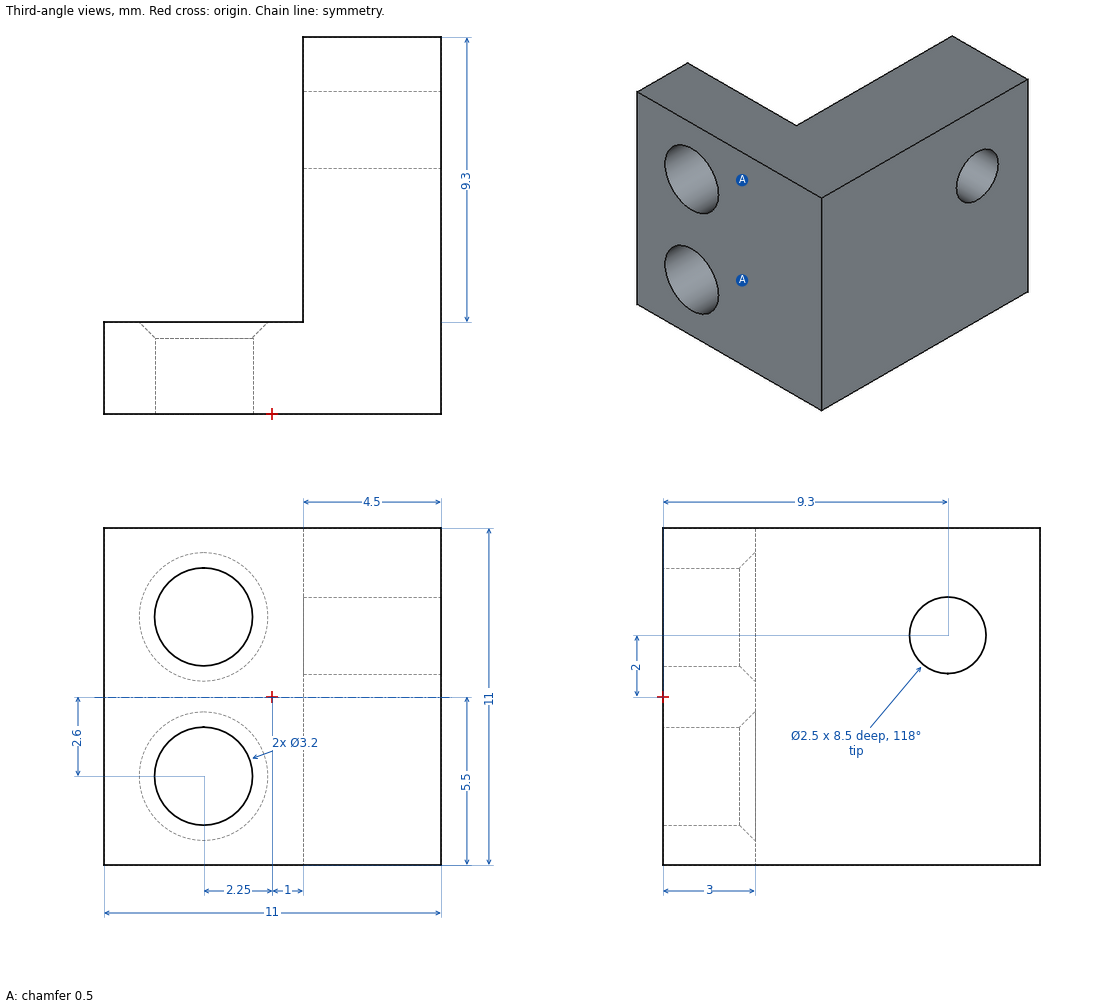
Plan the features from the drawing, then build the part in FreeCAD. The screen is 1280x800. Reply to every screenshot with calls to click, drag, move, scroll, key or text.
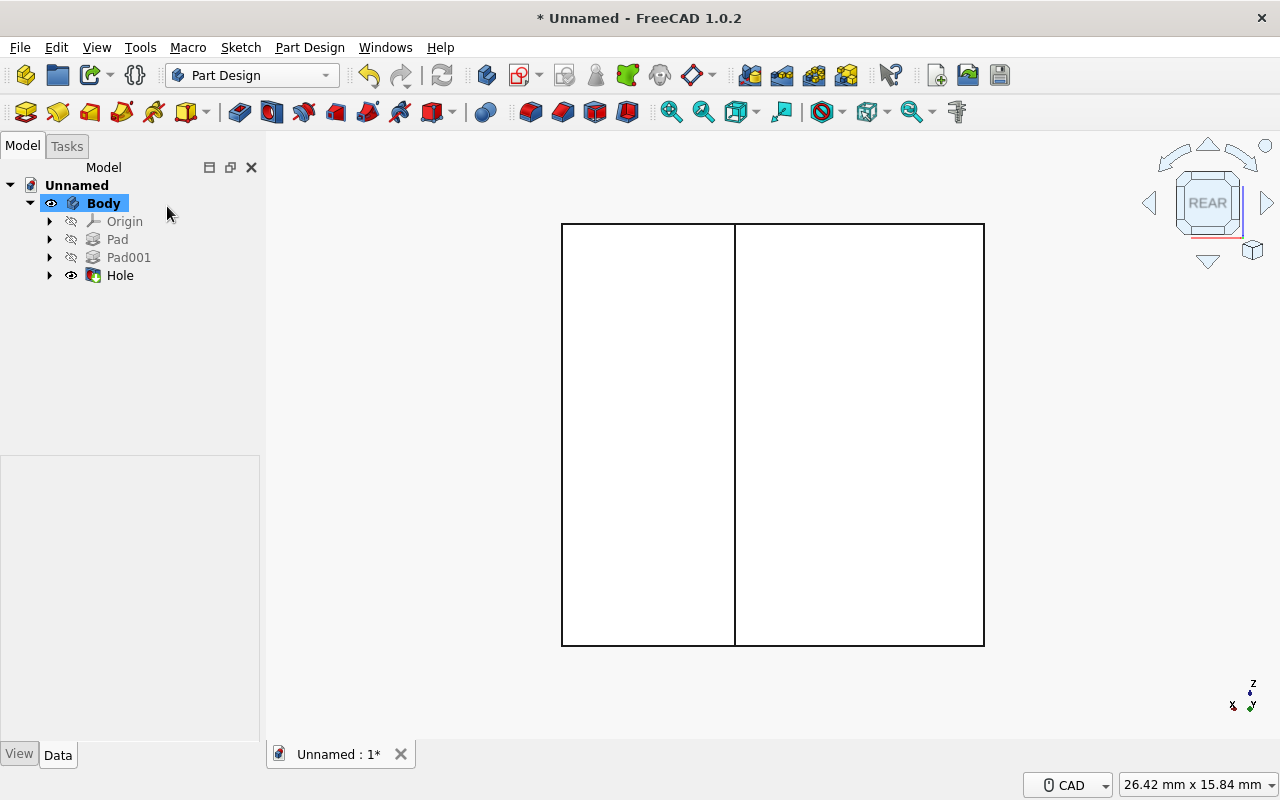
click(859, 374)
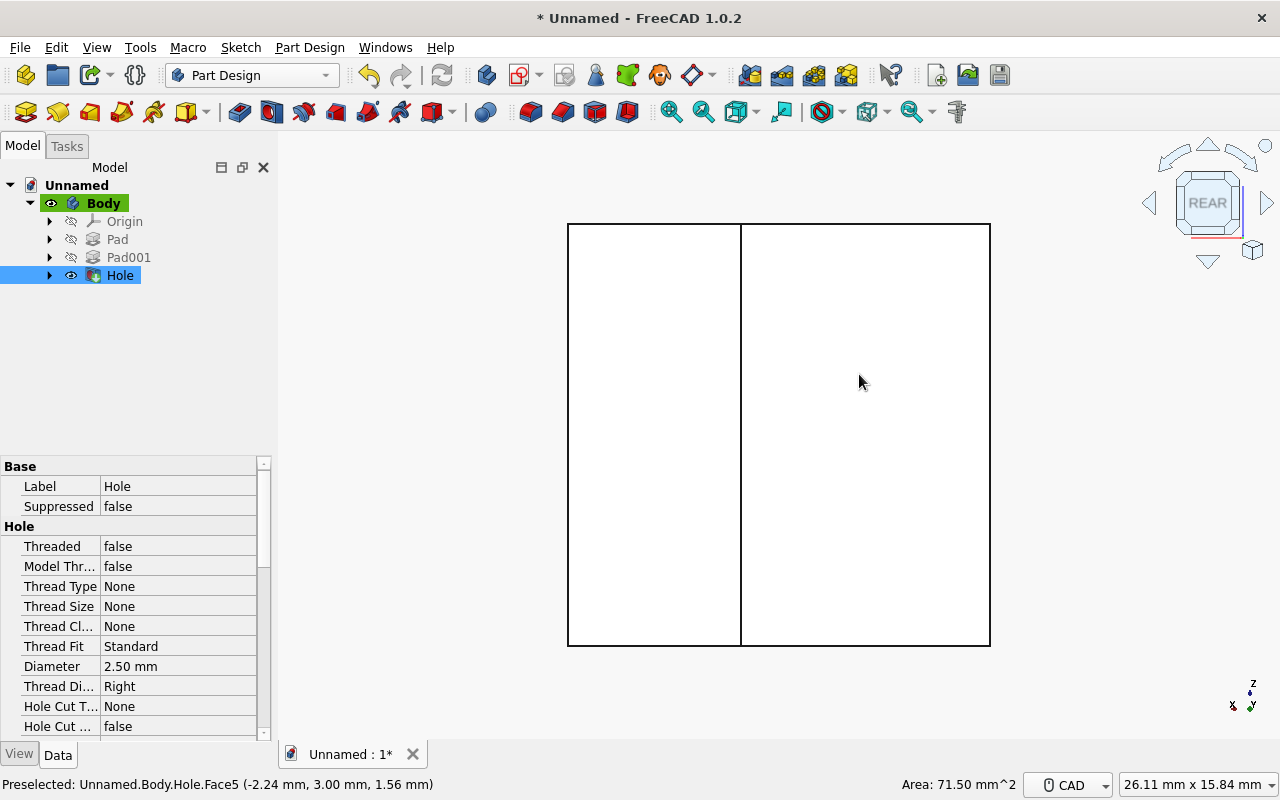
click(520, 76)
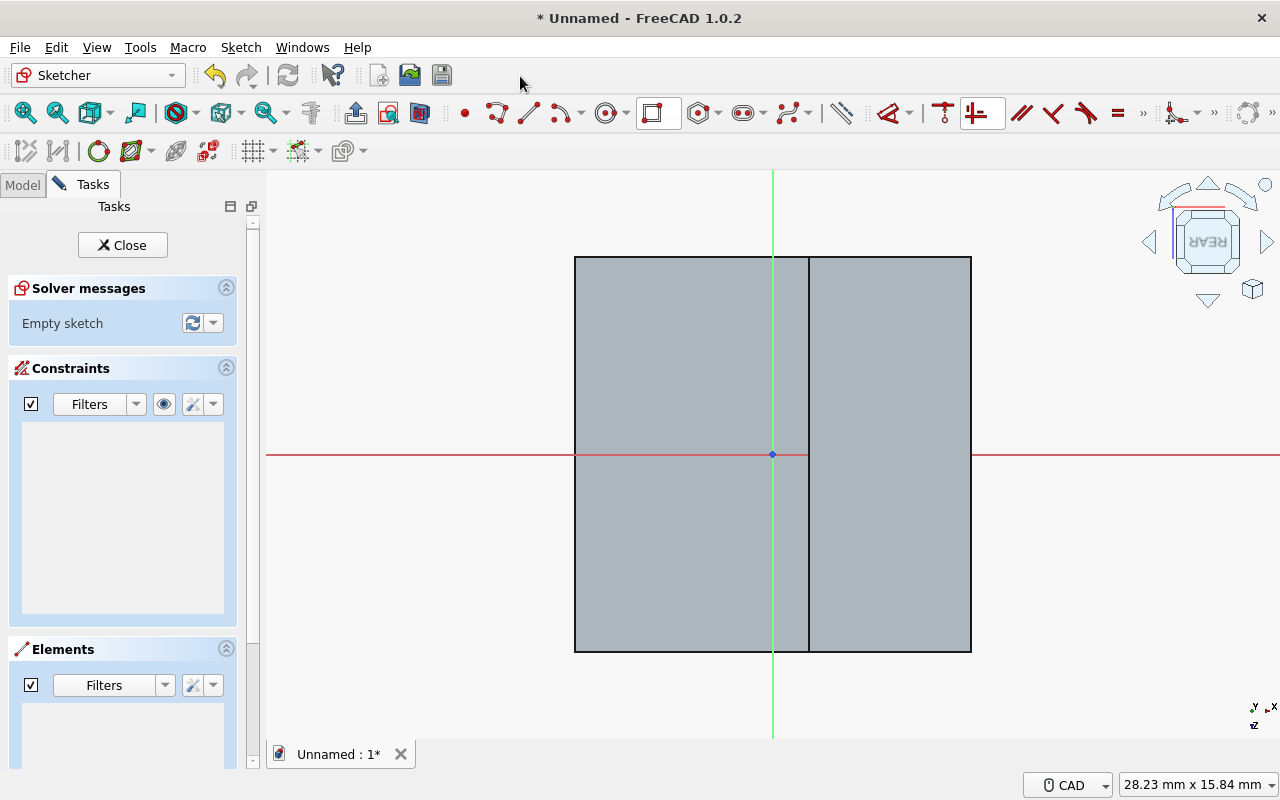
click(606, 114)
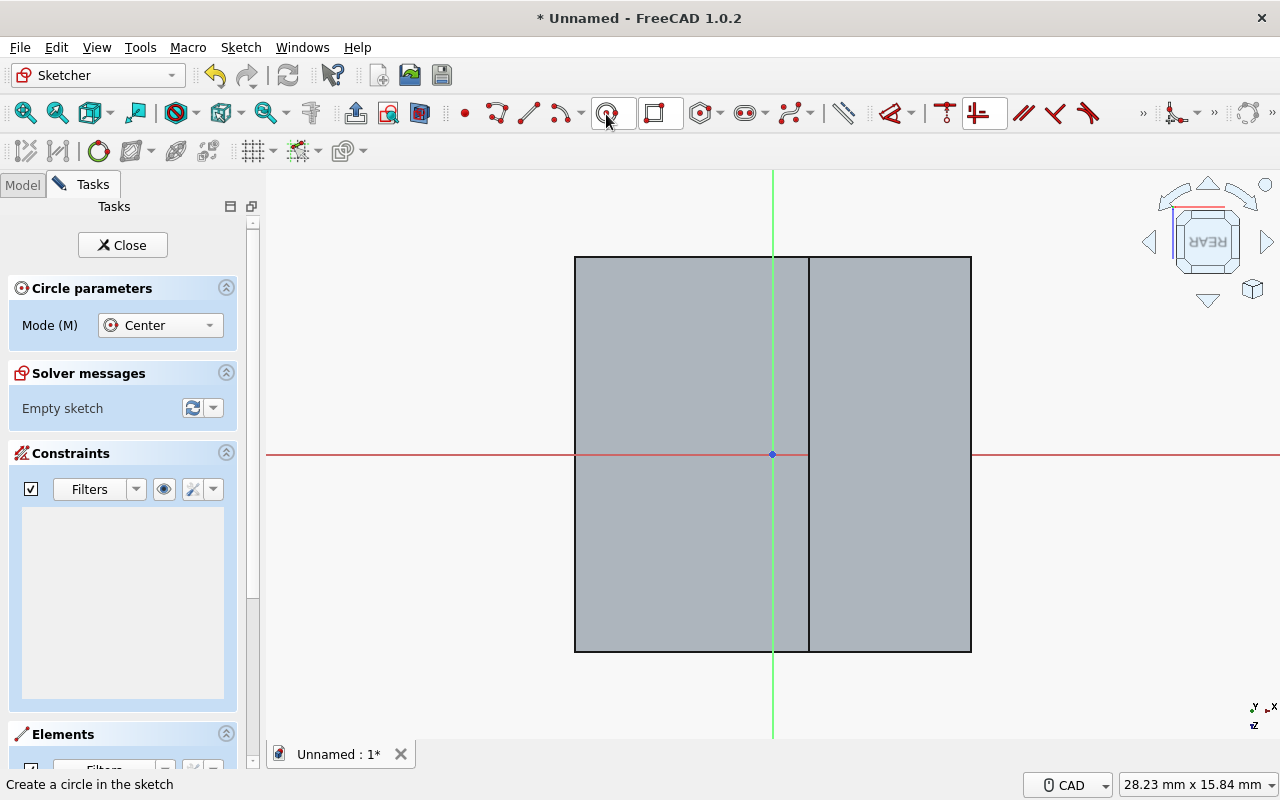
click(692, 361)
click(733, 320)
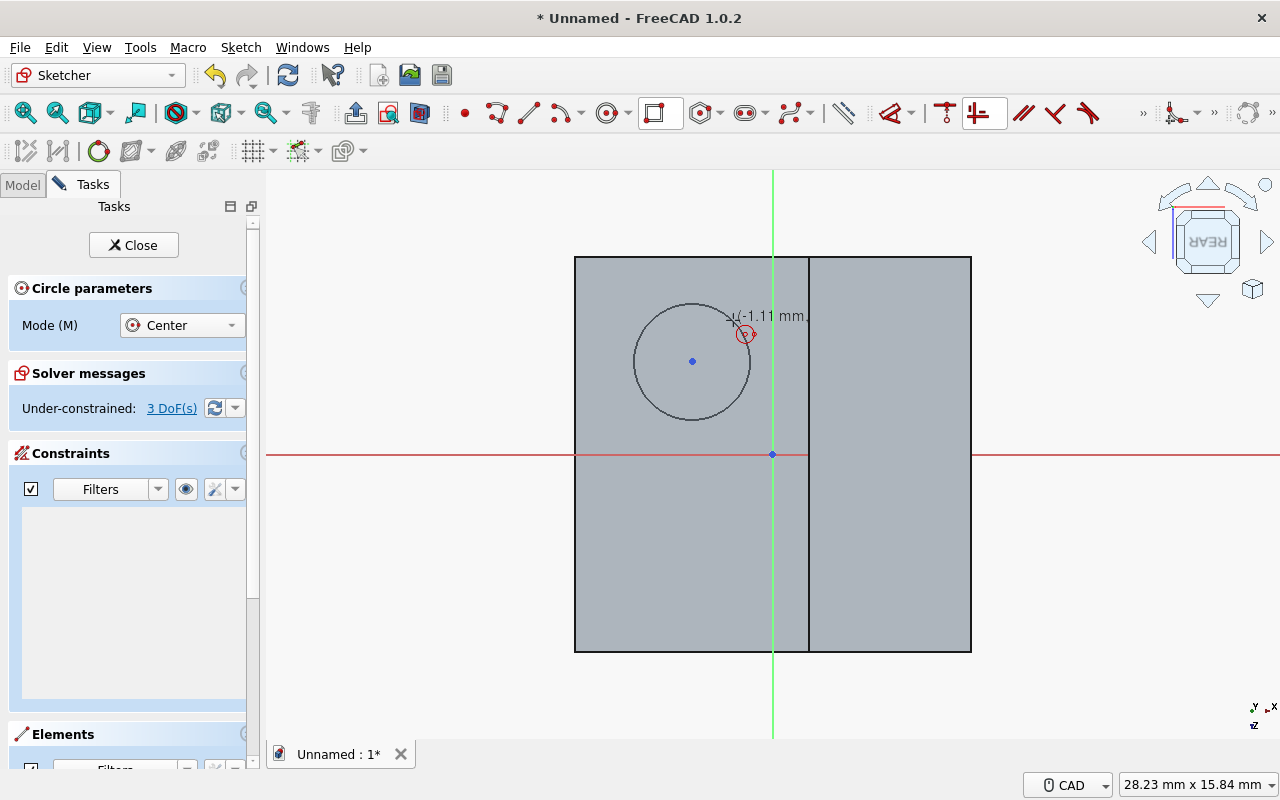
click(692, 548)
click(733, 507)
key(Escape)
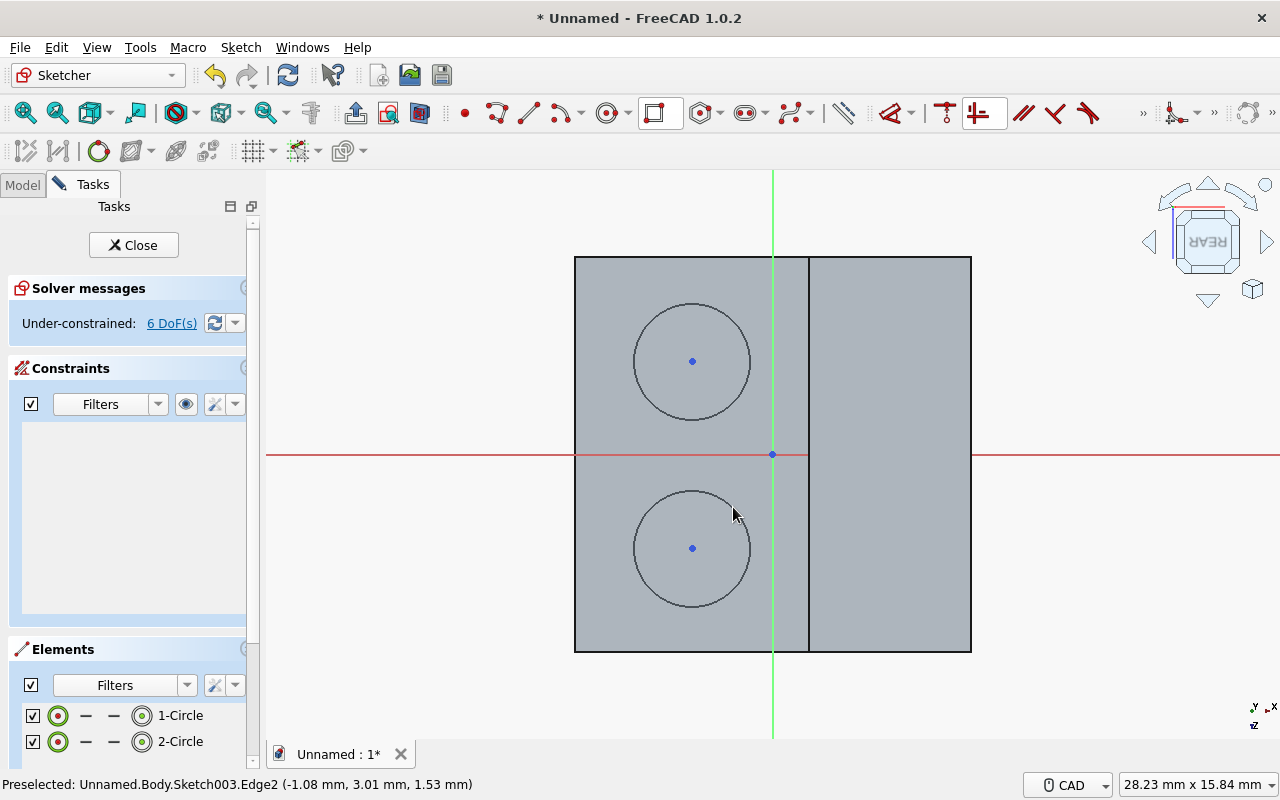
click(733, 321)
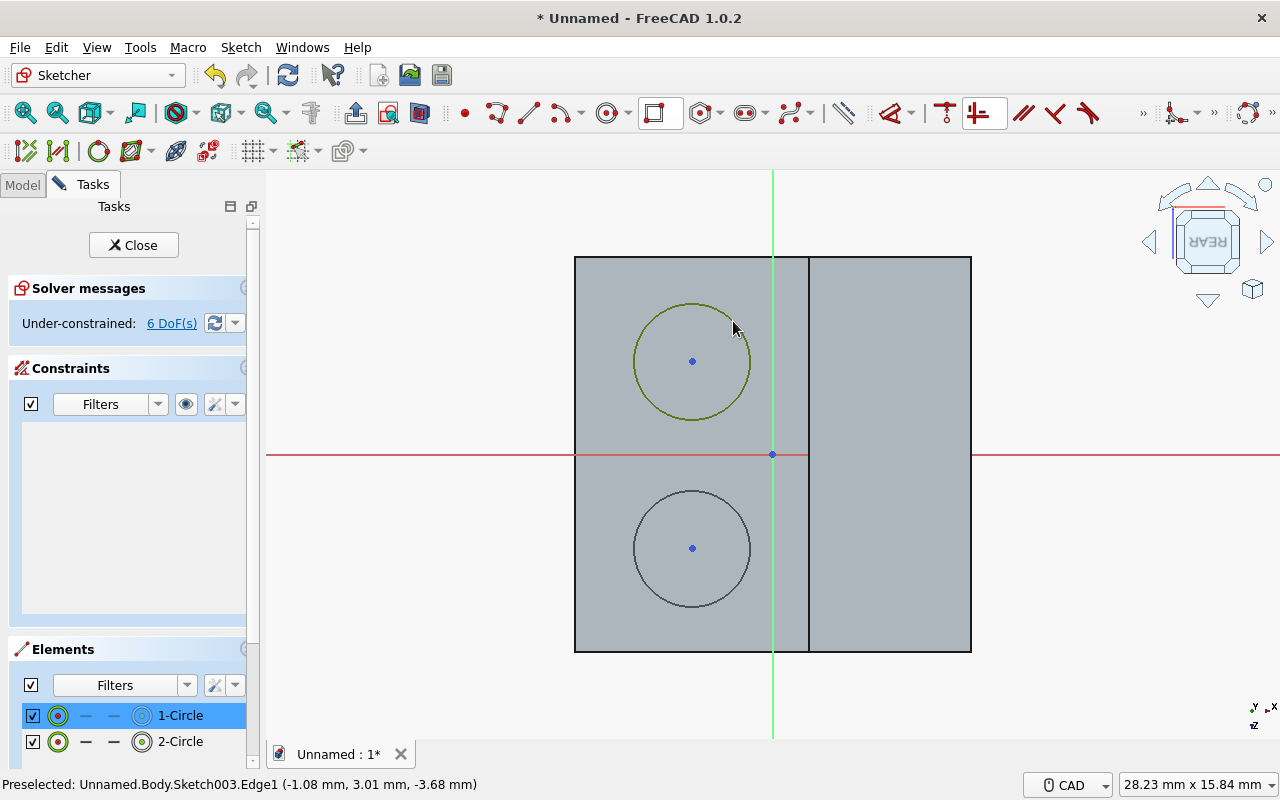
click(733, 508)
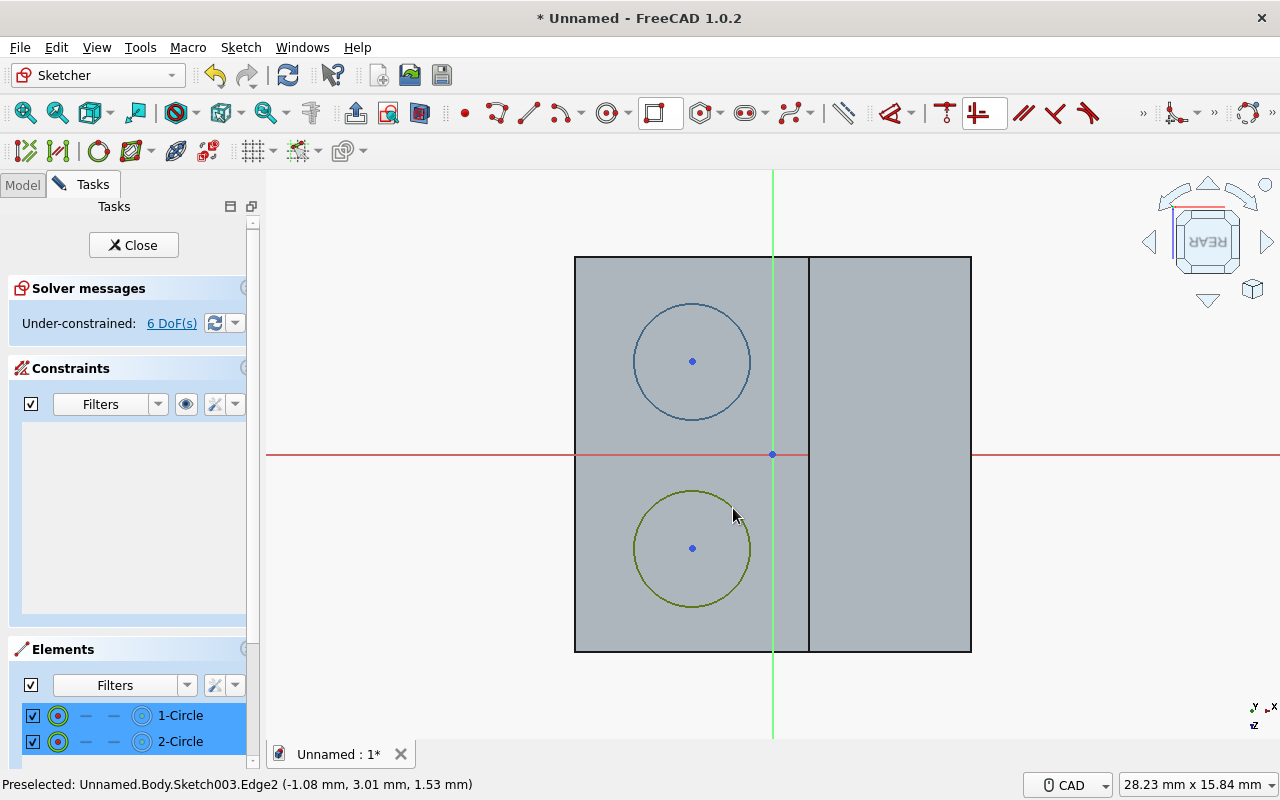
key(e)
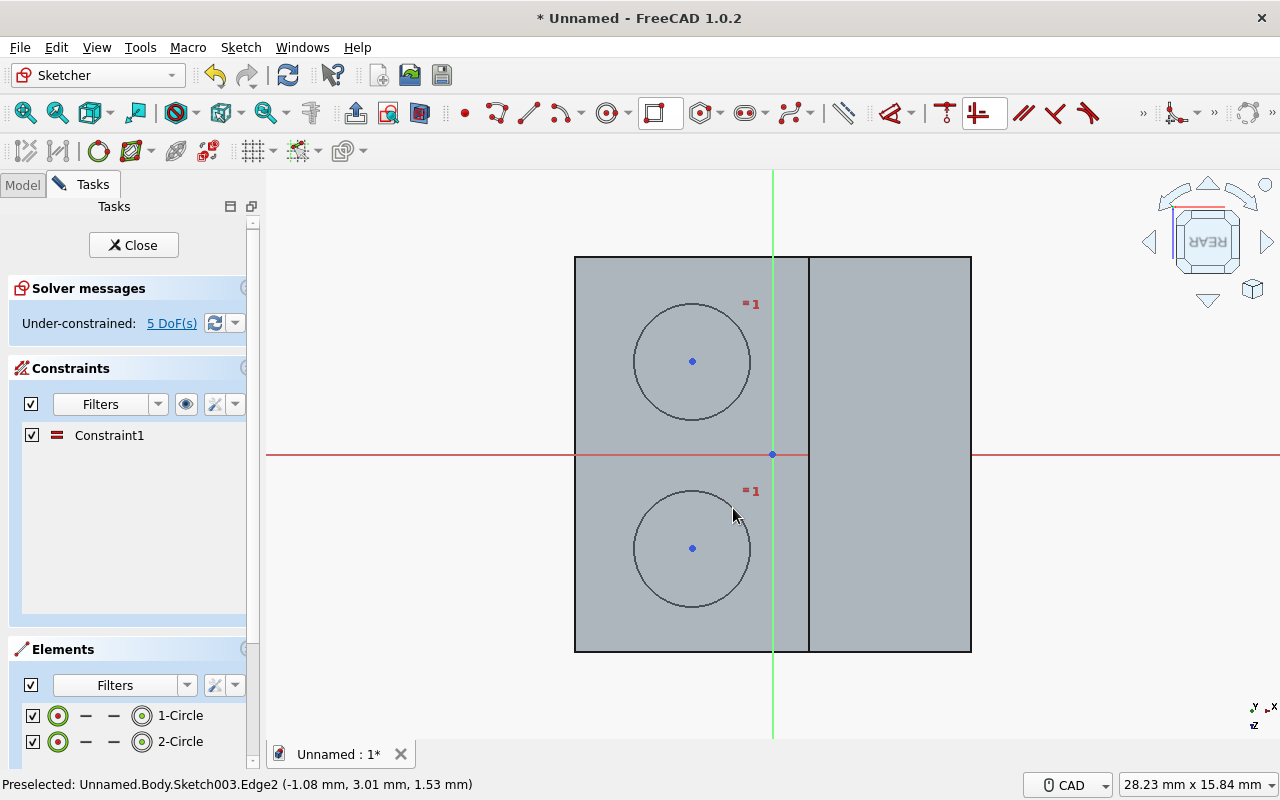
click(692, 362)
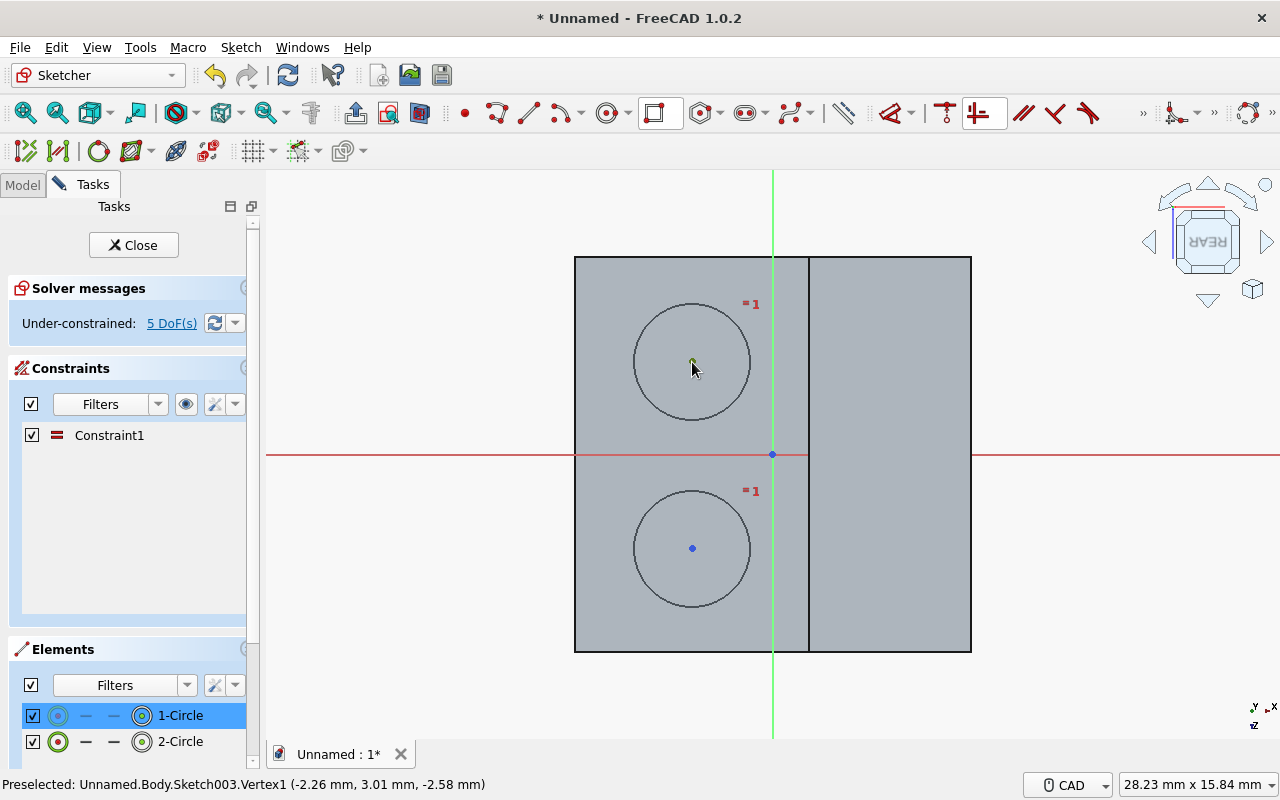
click(692, 549)